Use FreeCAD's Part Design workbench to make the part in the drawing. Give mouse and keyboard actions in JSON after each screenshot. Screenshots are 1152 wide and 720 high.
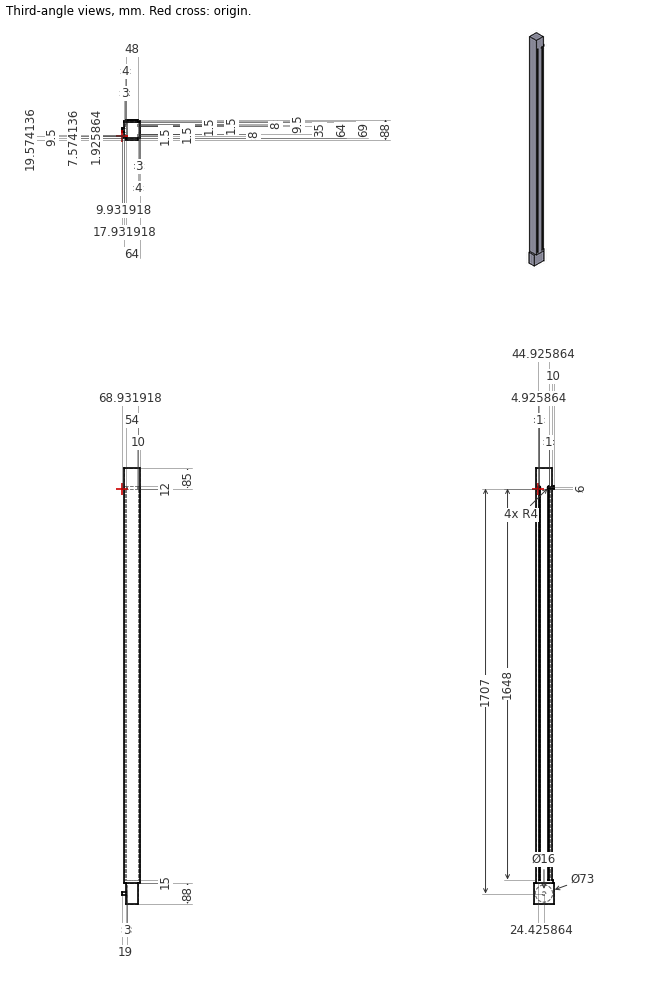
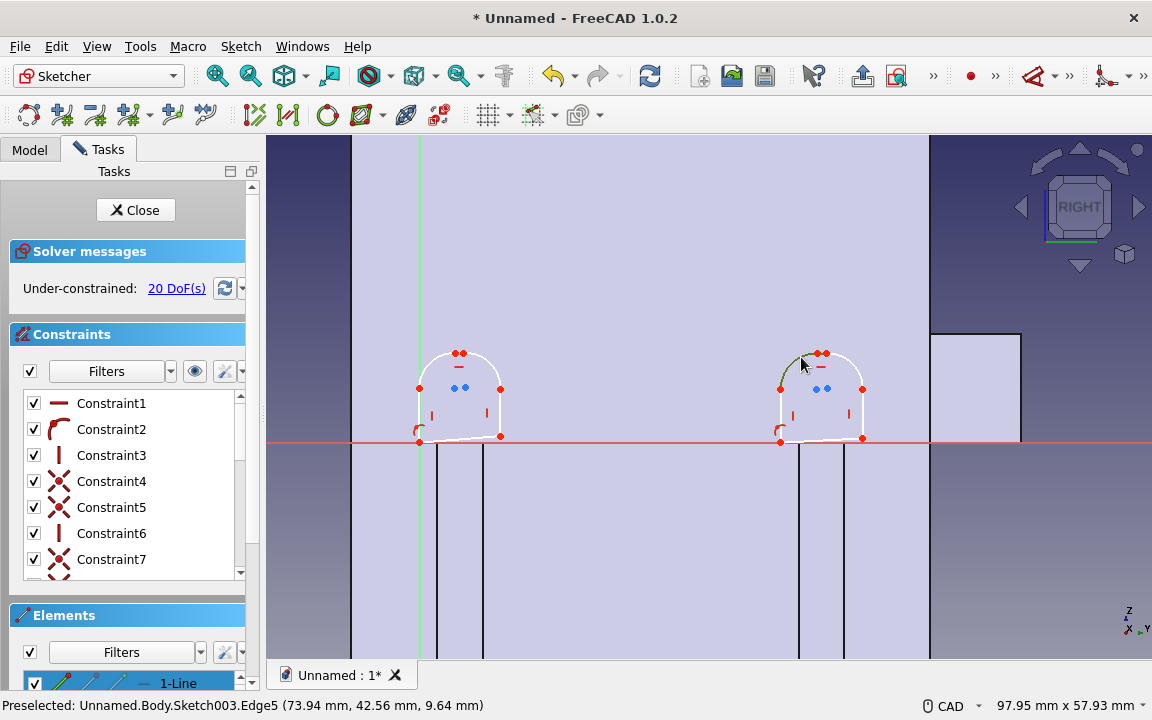
{"action": "key", "text": "t"}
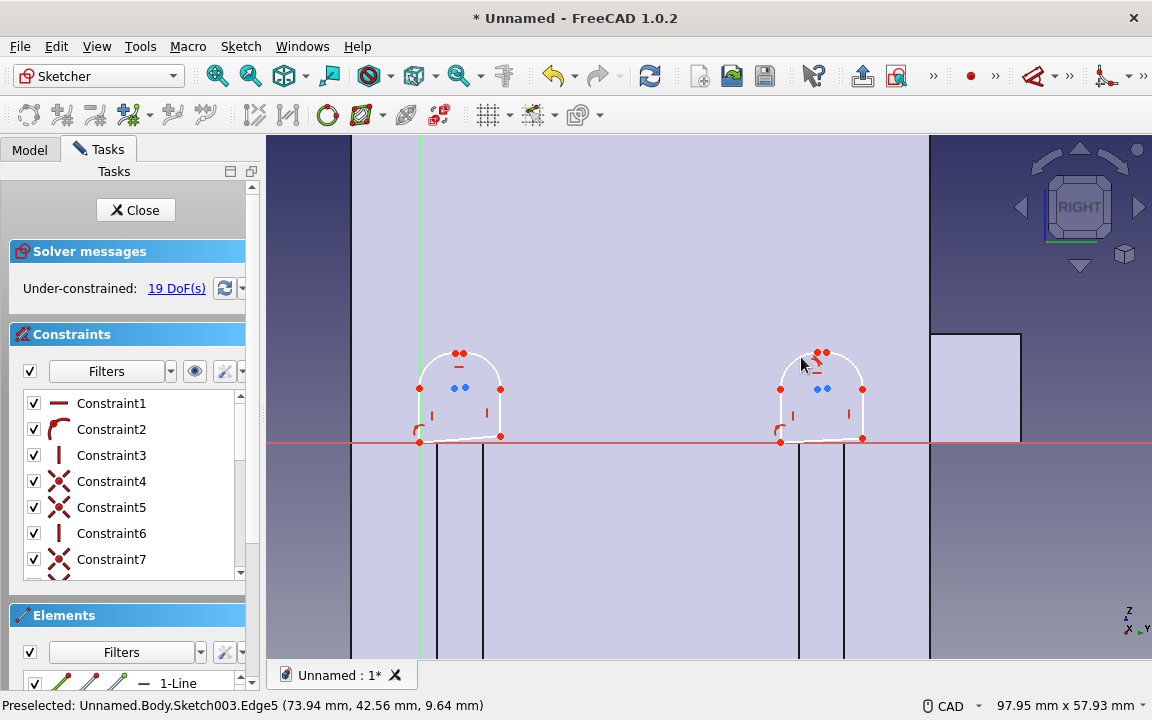
{"action": "scroll", "coordinate": [822, 353], "scroll_direction": "up", "scroll_amount": 6}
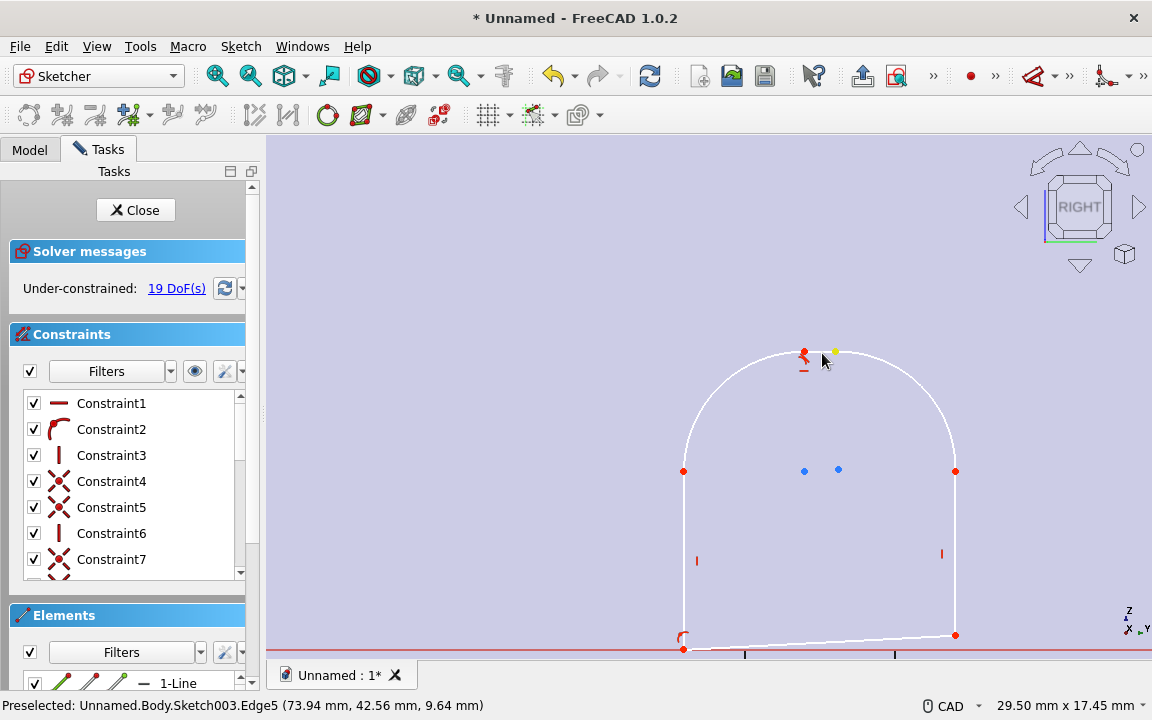
{"action": "left_click", "coordinate": [820, 352]}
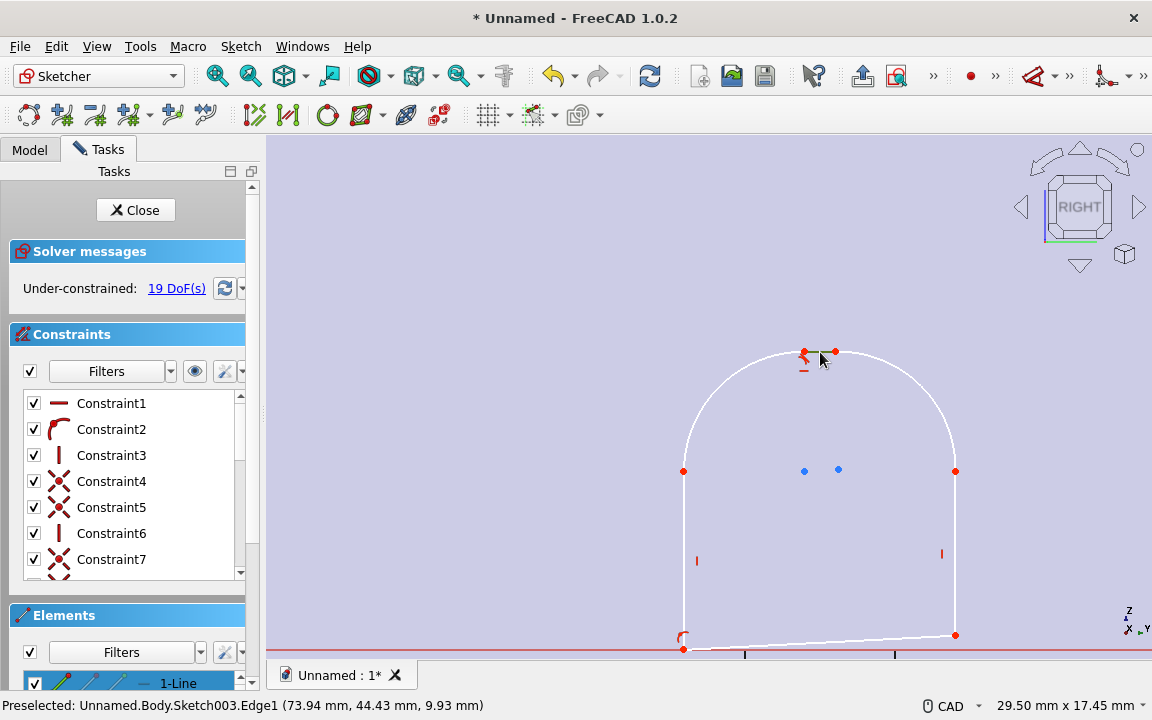
{"action": "left_click", "coordinate": [943, 417]}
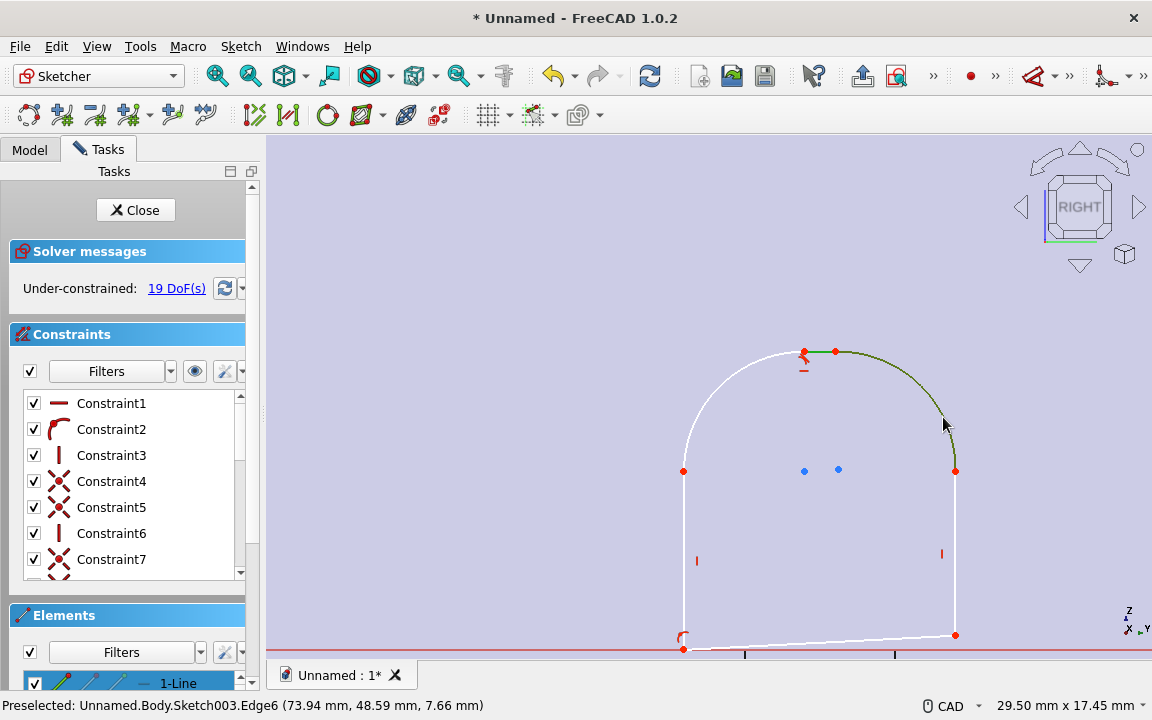
{"action": "key", "text": "t"}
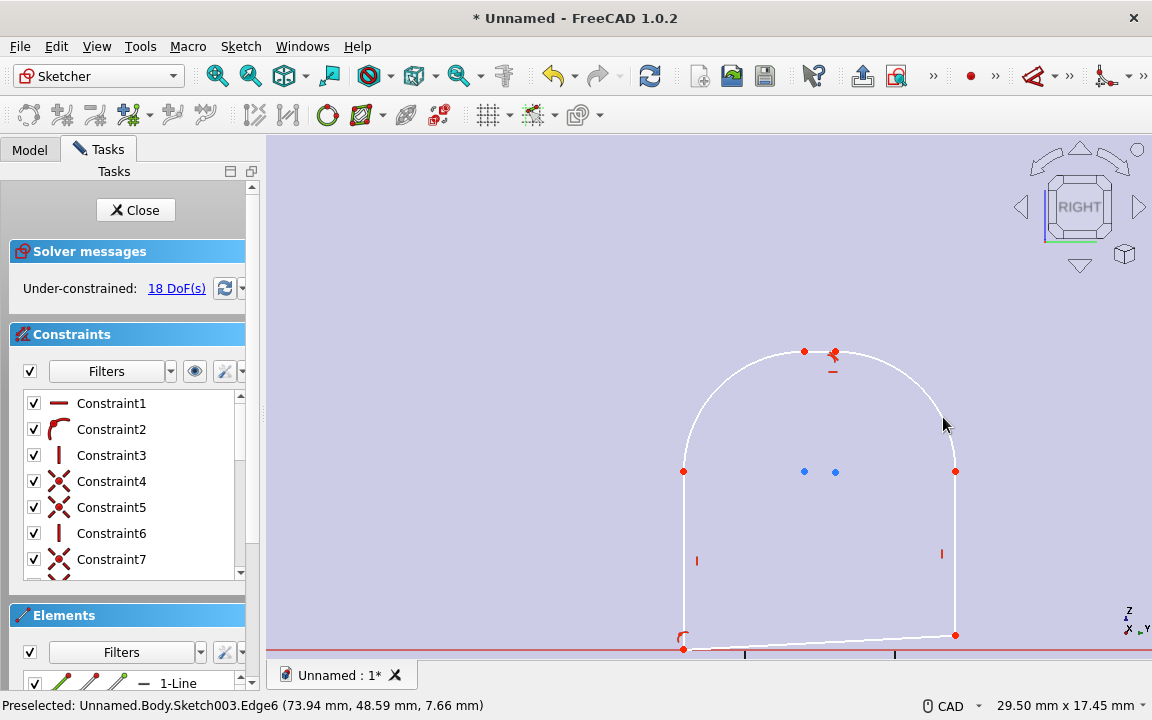
{"action": "left_click", "coordinate": [684, 525]}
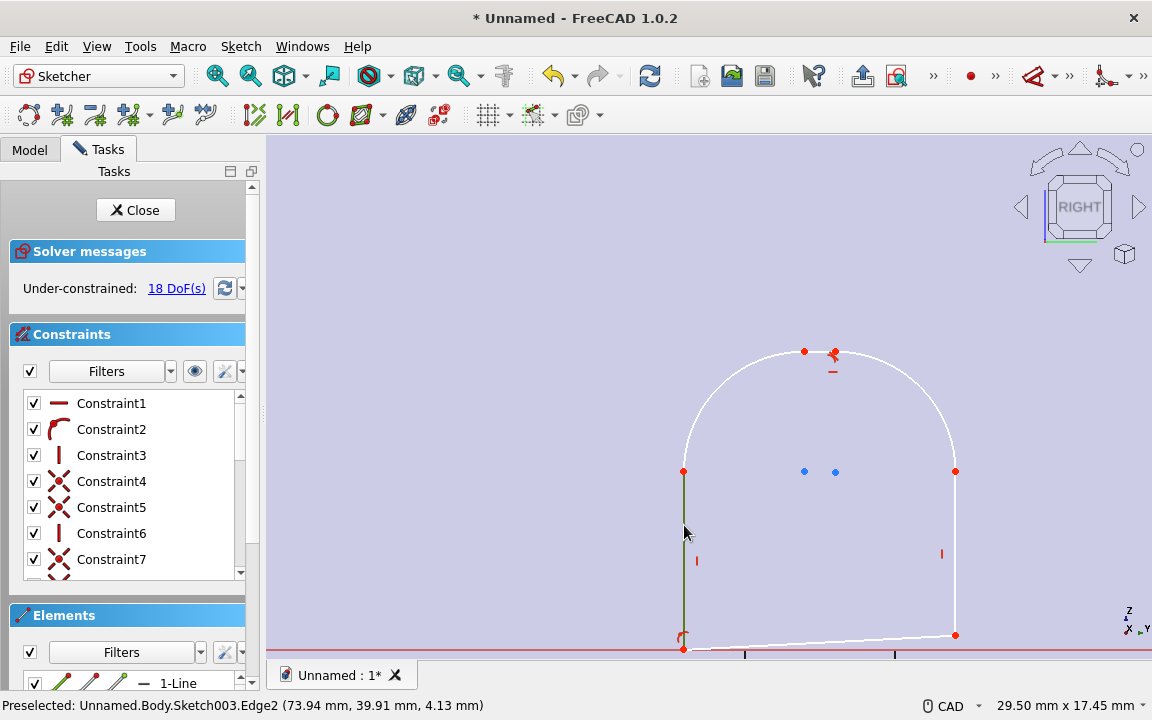
{"action": "left_click", "coordinate": [750, 365]}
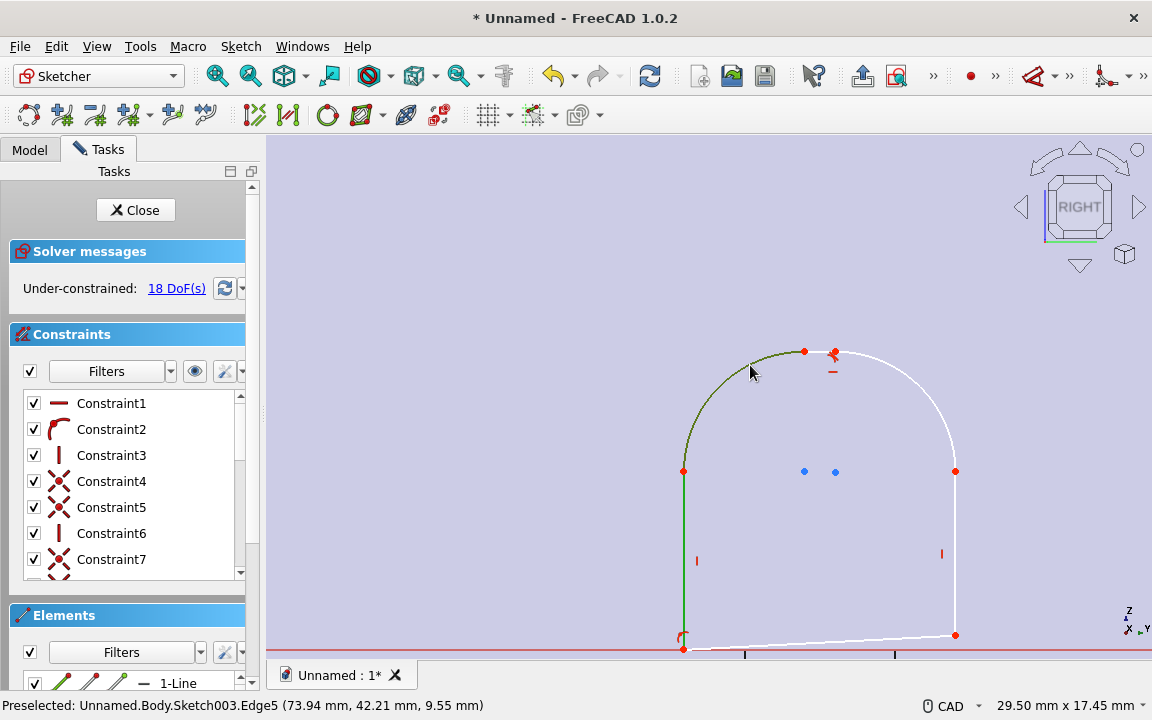
{"action": "key", "text": "t"}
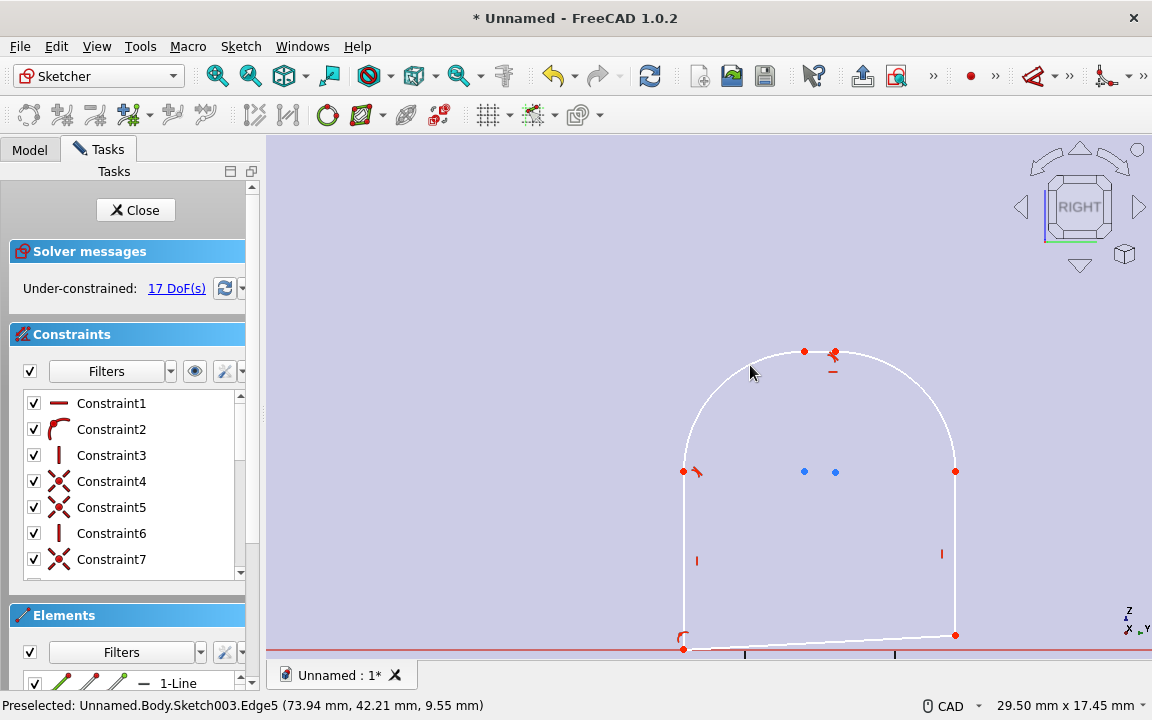
{"action": "left_click", "coordinate": [955, 586]}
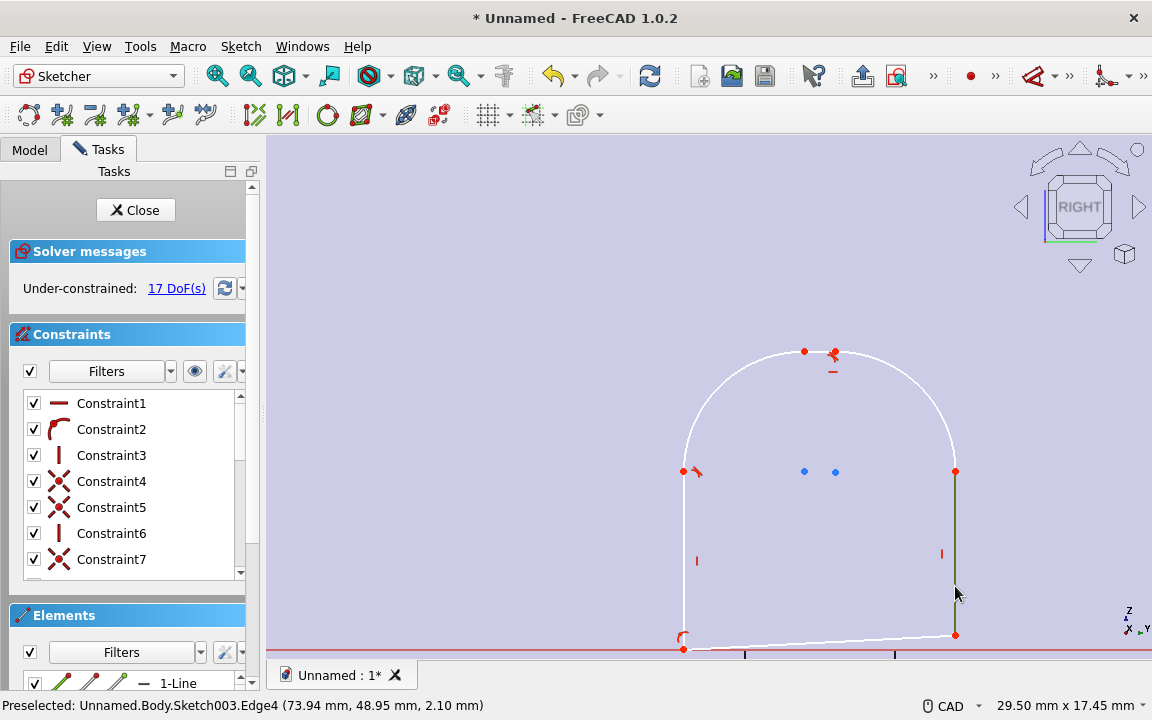
{"action": "left_click", "coordinate": [942, 417]}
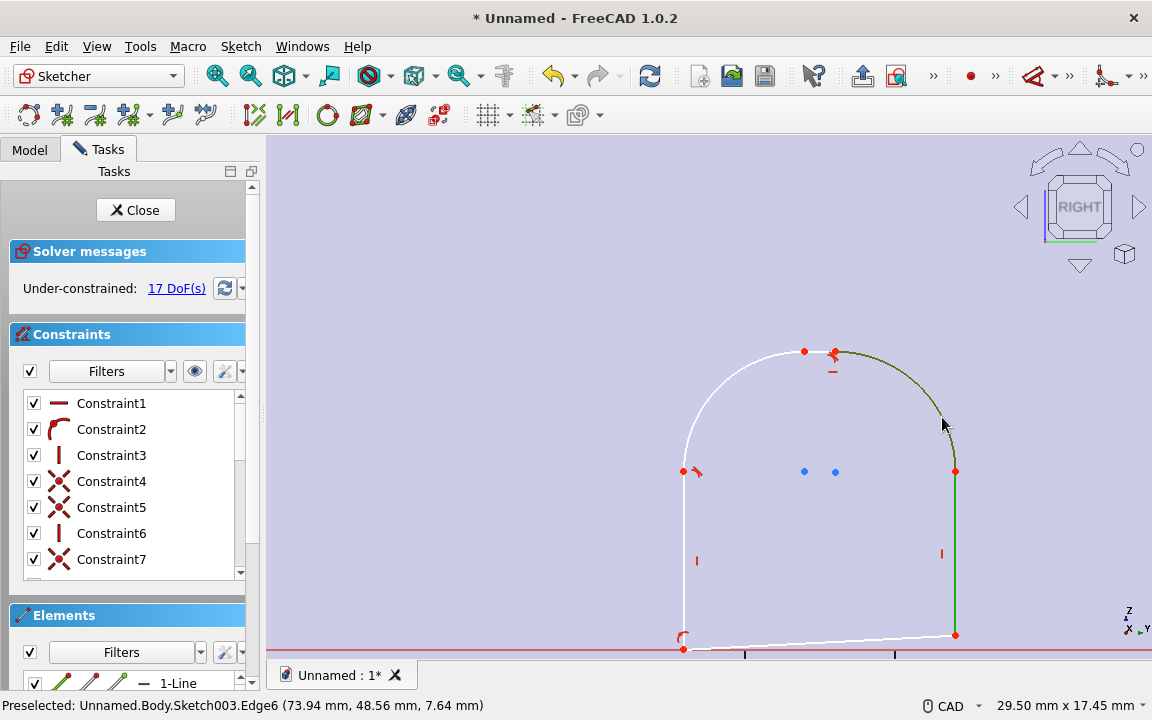
{"action": "key", "text": "t"}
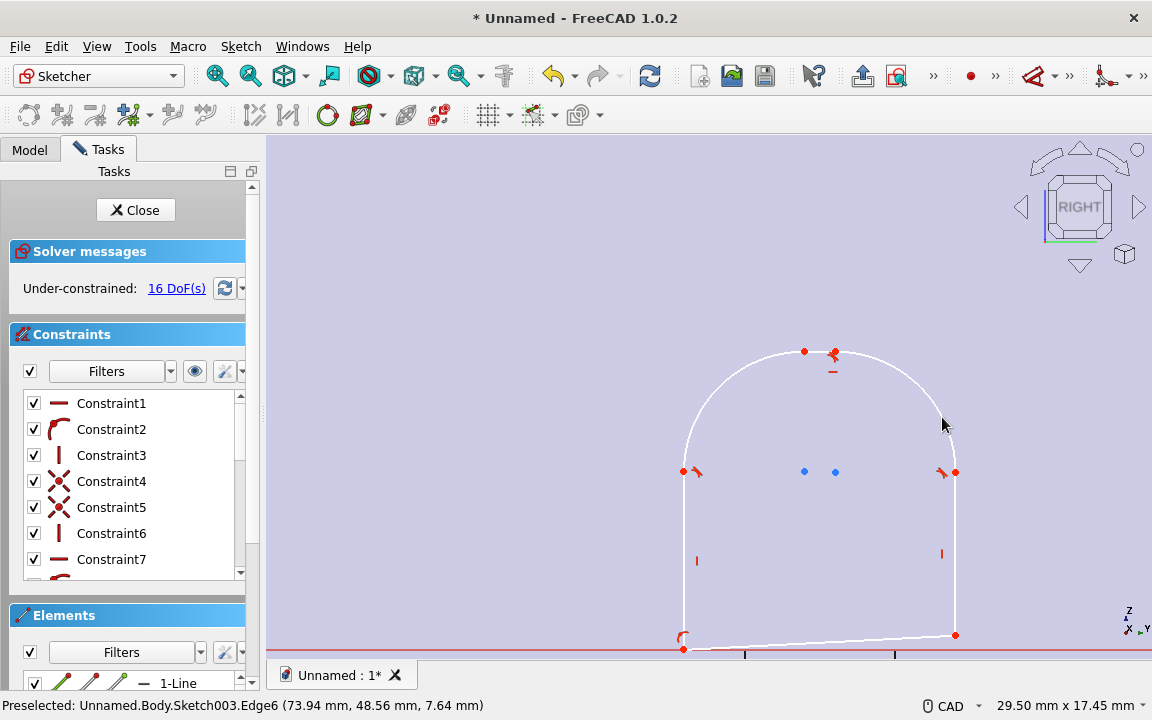
{"action": "scroll", "coordinate": [822, 353], "scroll_direction": "down", "scroll_amount": 6}